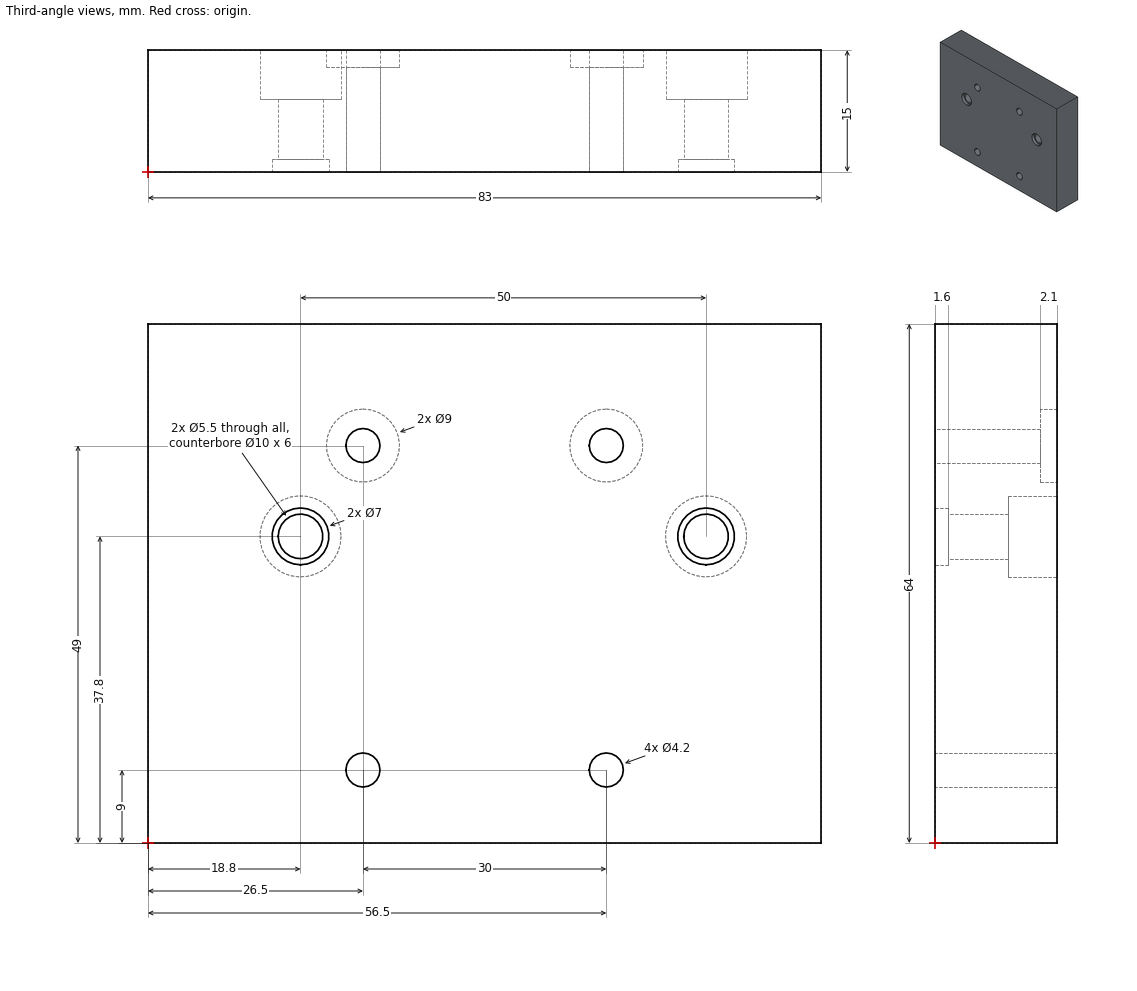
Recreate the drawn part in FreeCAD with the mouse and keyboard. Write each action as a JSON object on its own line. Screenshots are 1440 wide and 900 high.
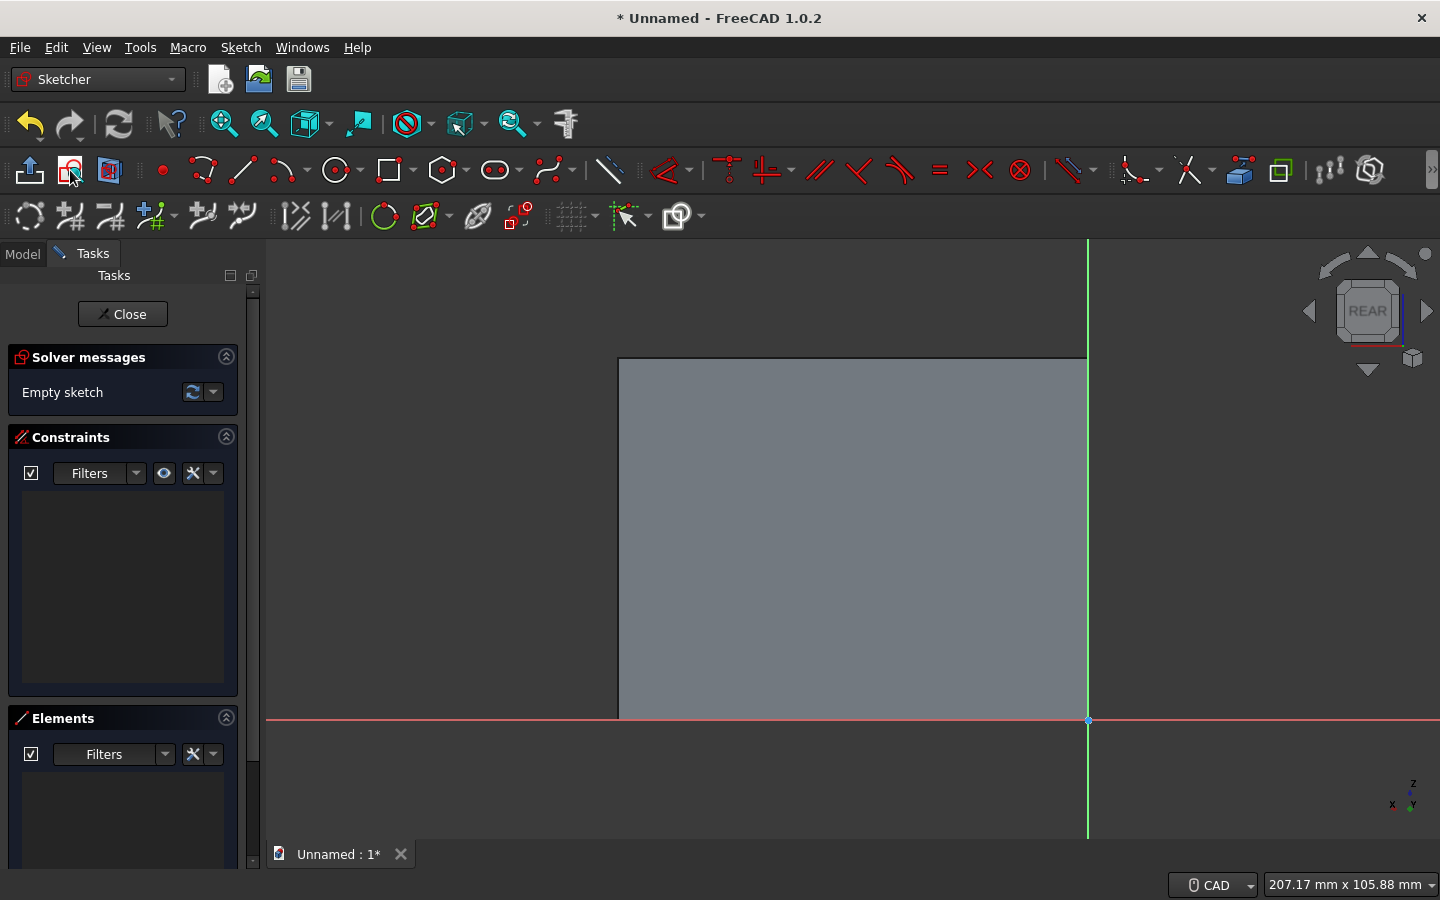
{"action": "scroll", "coordinate": [1008, 686], "scroll_direction": "up", "scroll_amount": 3}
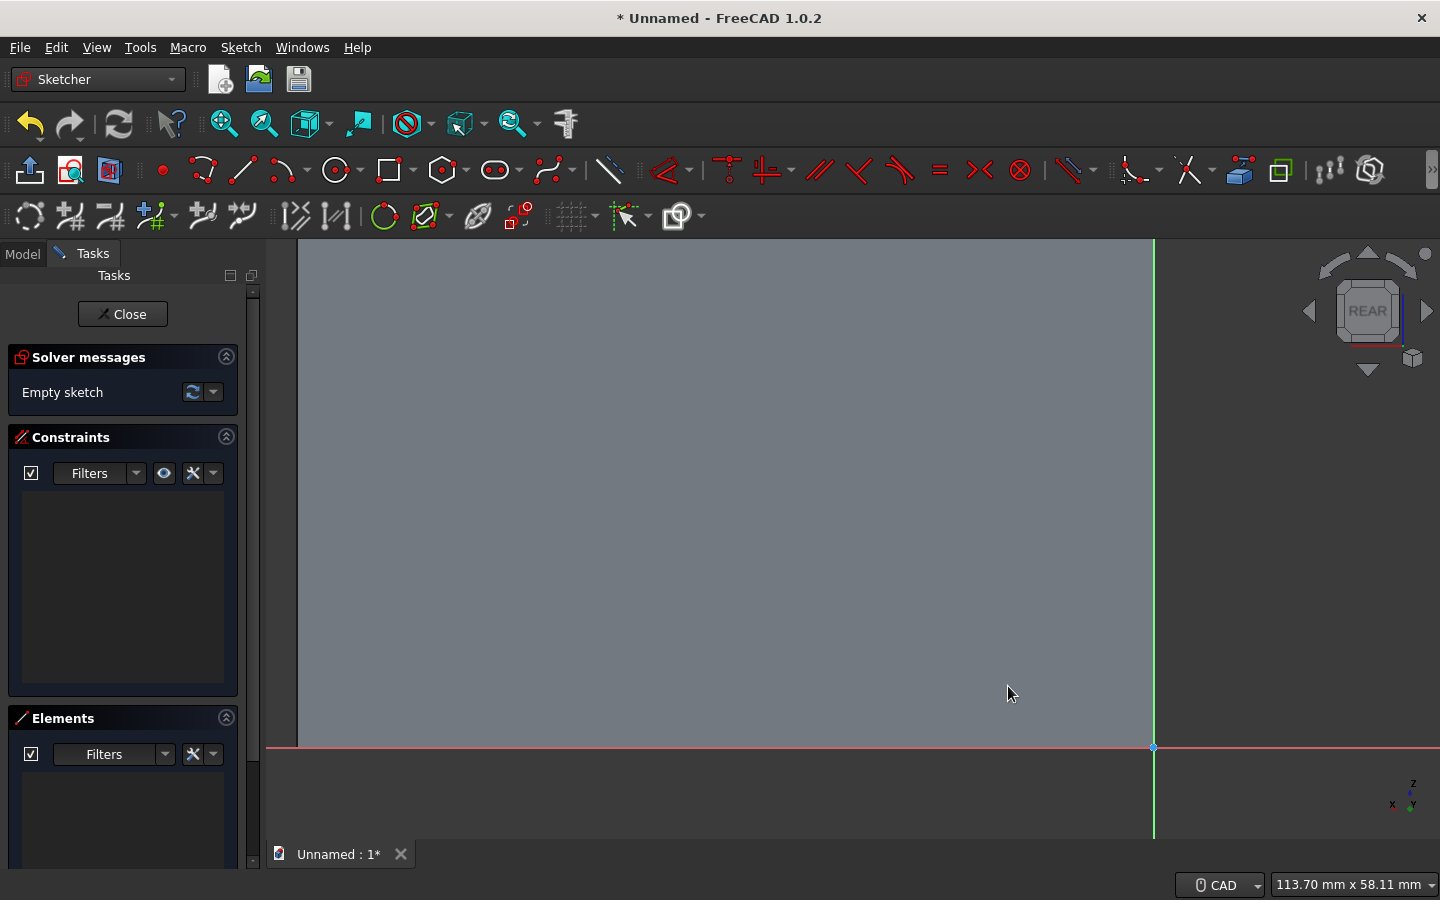
{"action": "left_click", "coordinate": [336, 170]}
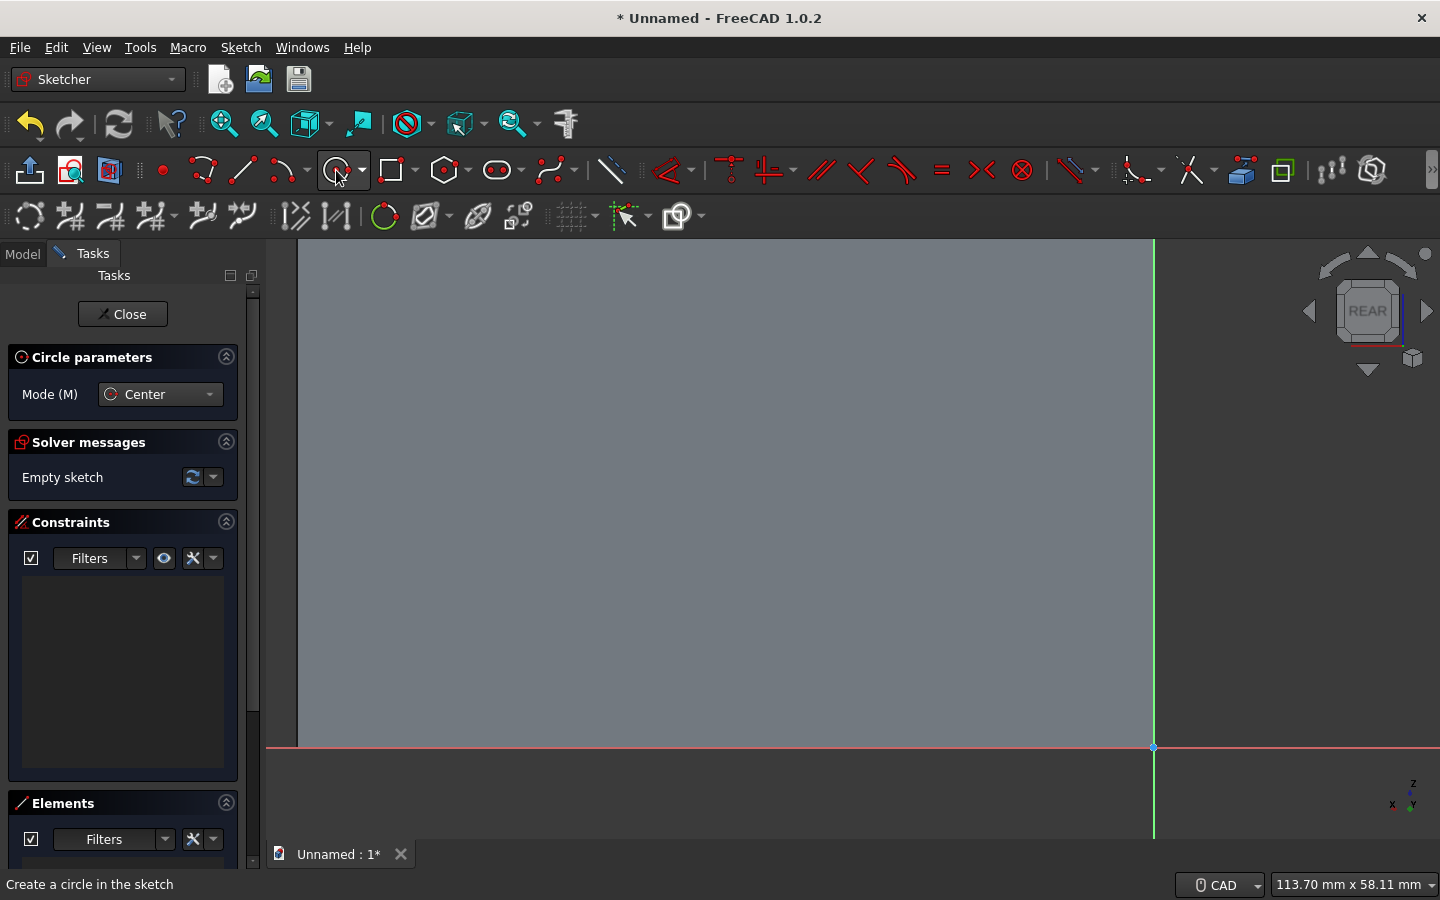
{"action": "left_click", "coordinate": [959, 358]}
{"action": "left_click", "coordinate": [980, 338]}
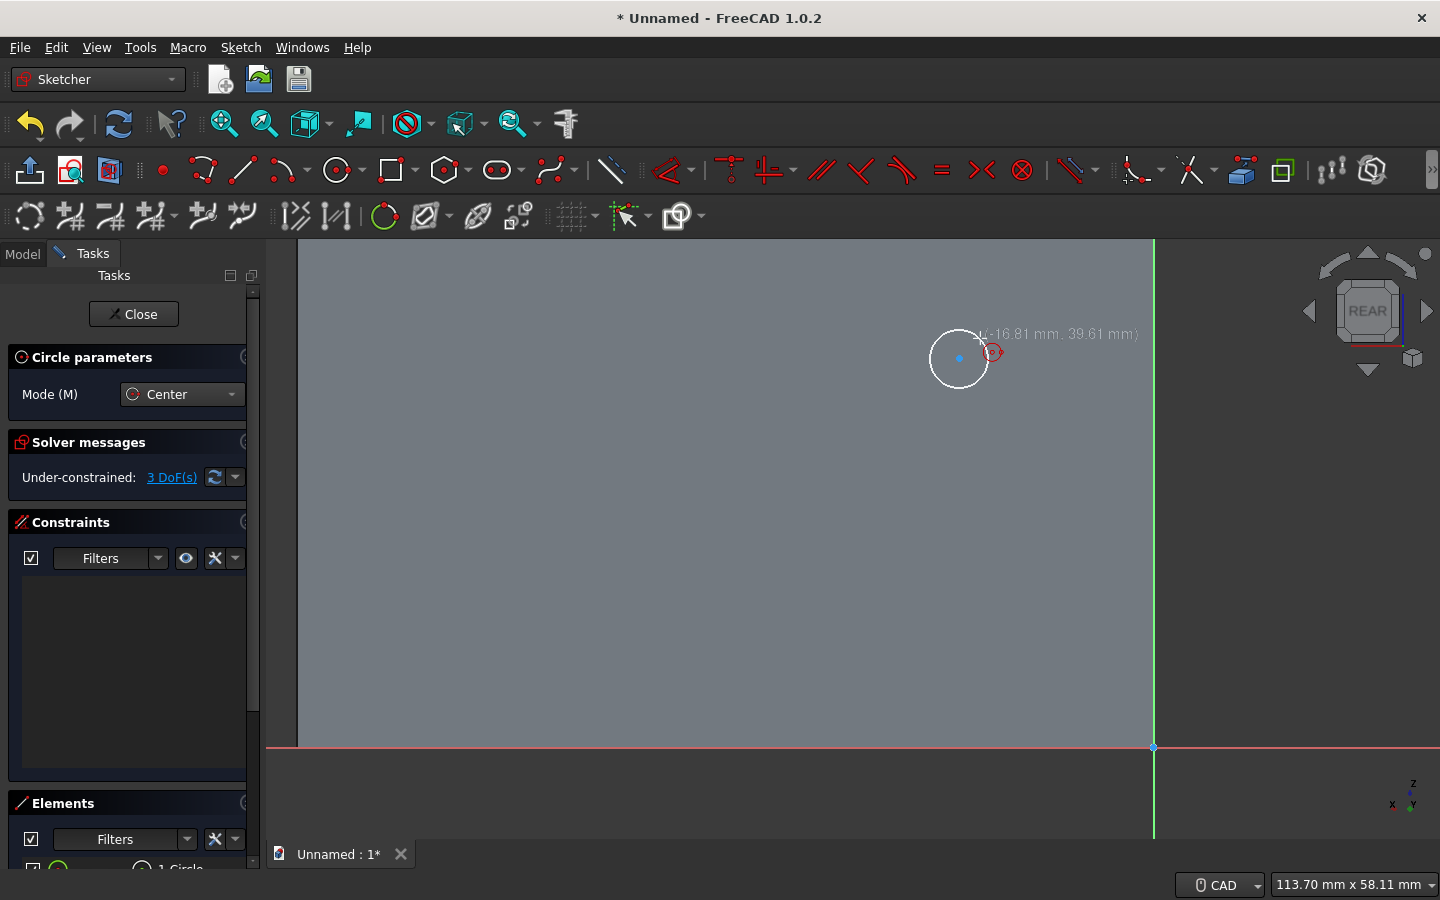
{"action": "left_click", "coordinate": [443, 358]}
{"action": "left_click", "coordinate": [463, 338]}
{"action": "key", "text": "Escape"}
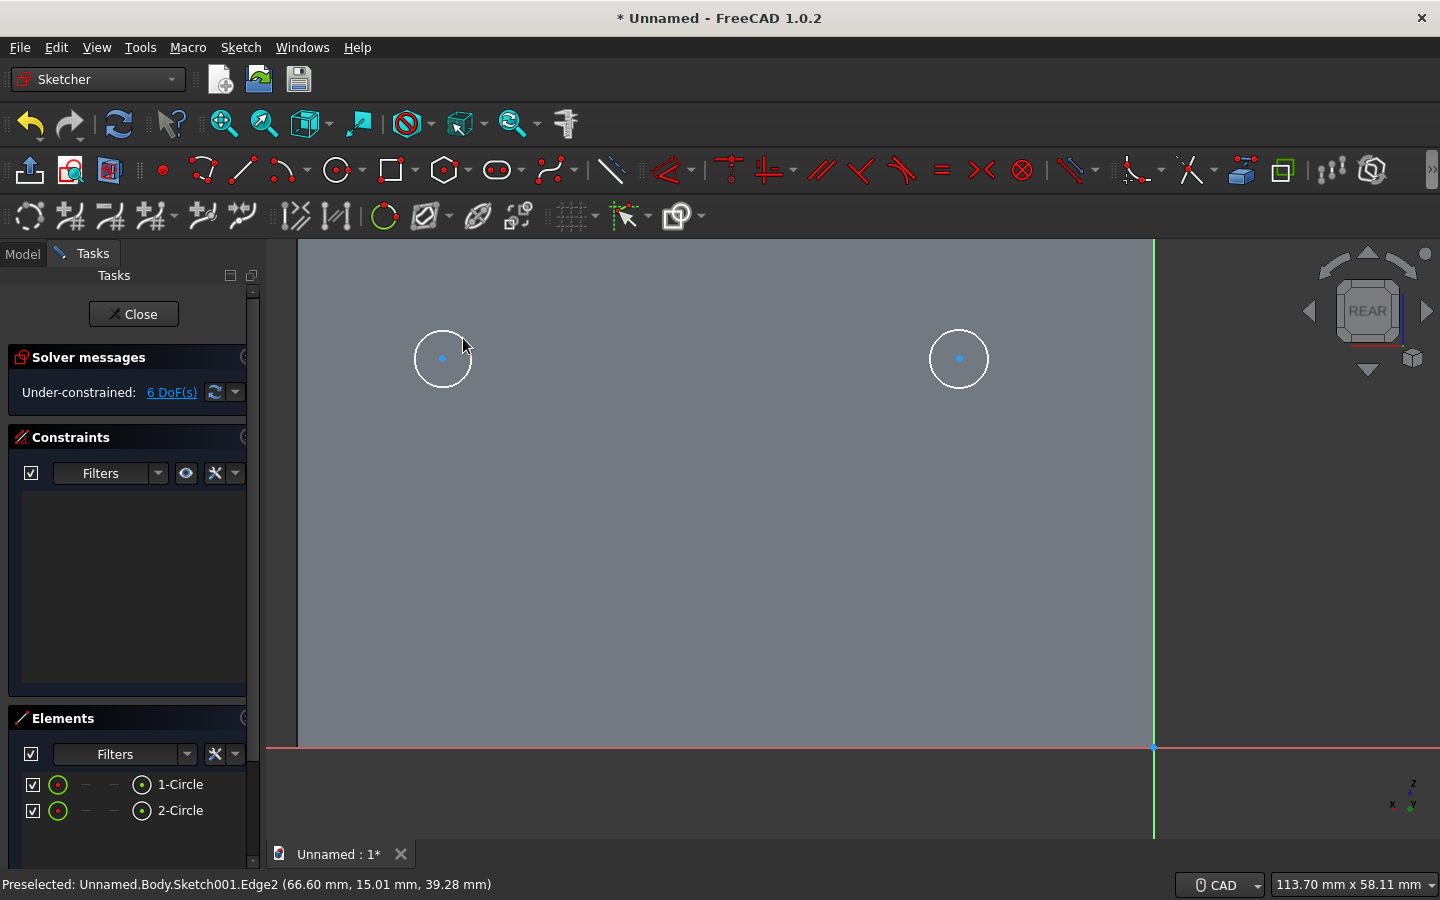
{"action": "left_click", "coordinate": [979, 338]}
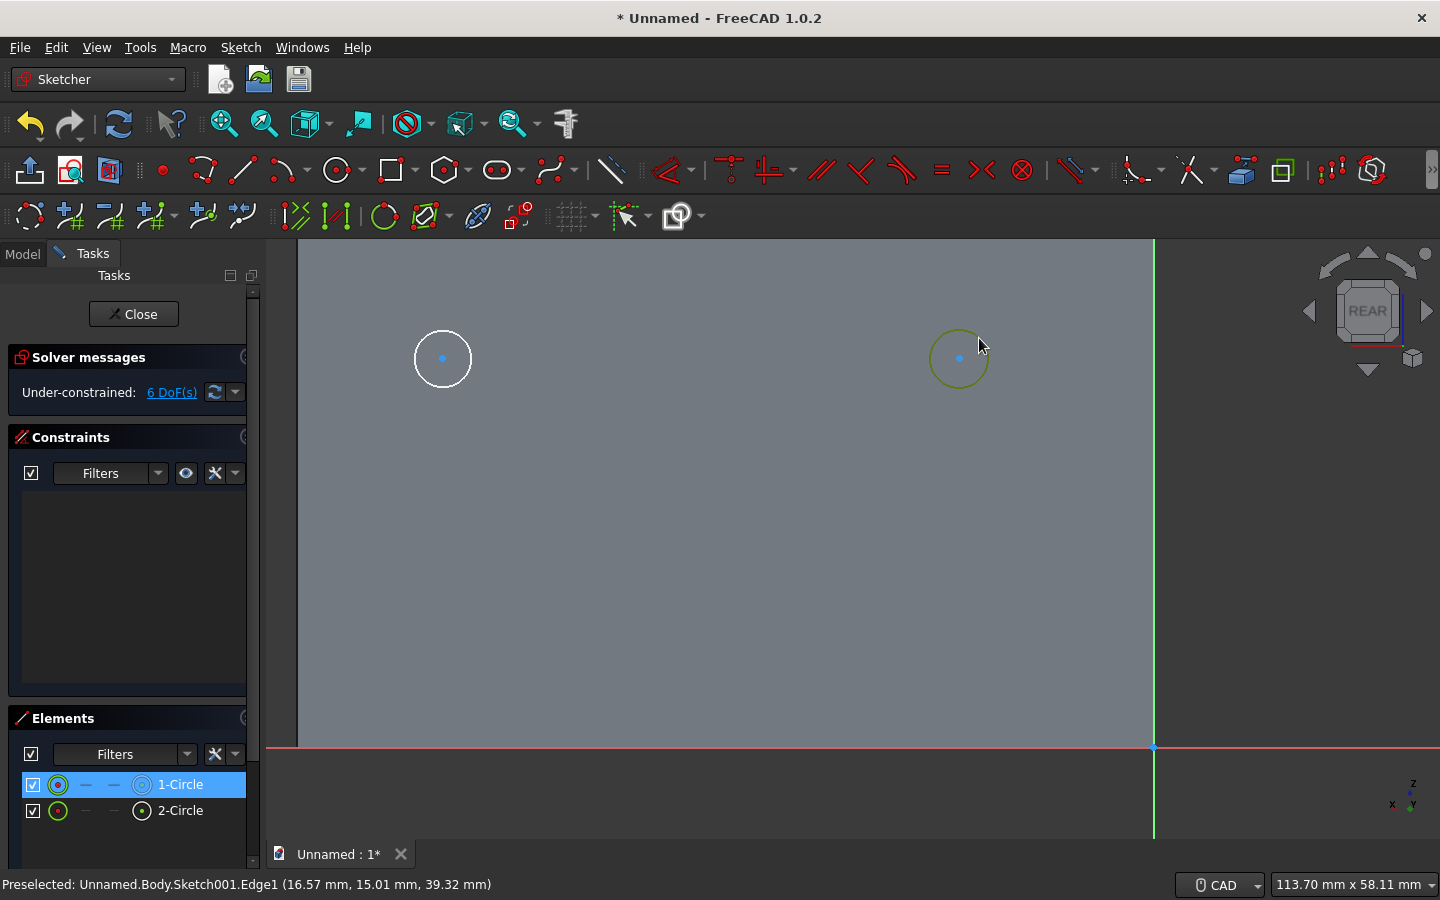
{"action": "left_click", "coordinate": [463, 339]}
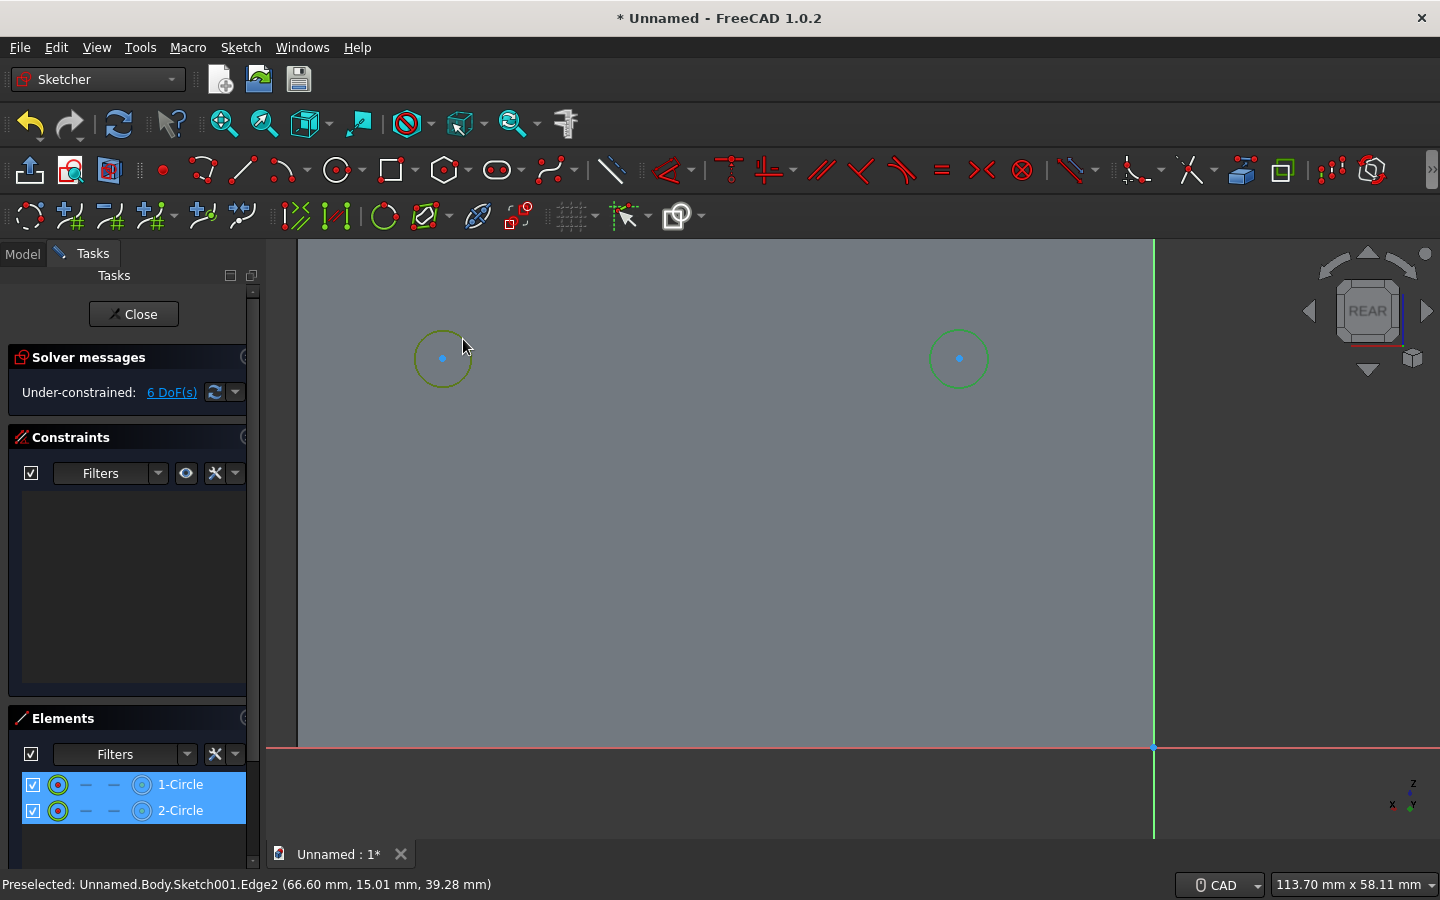
{"action": "left_click", "coordinate": [942, 170]}